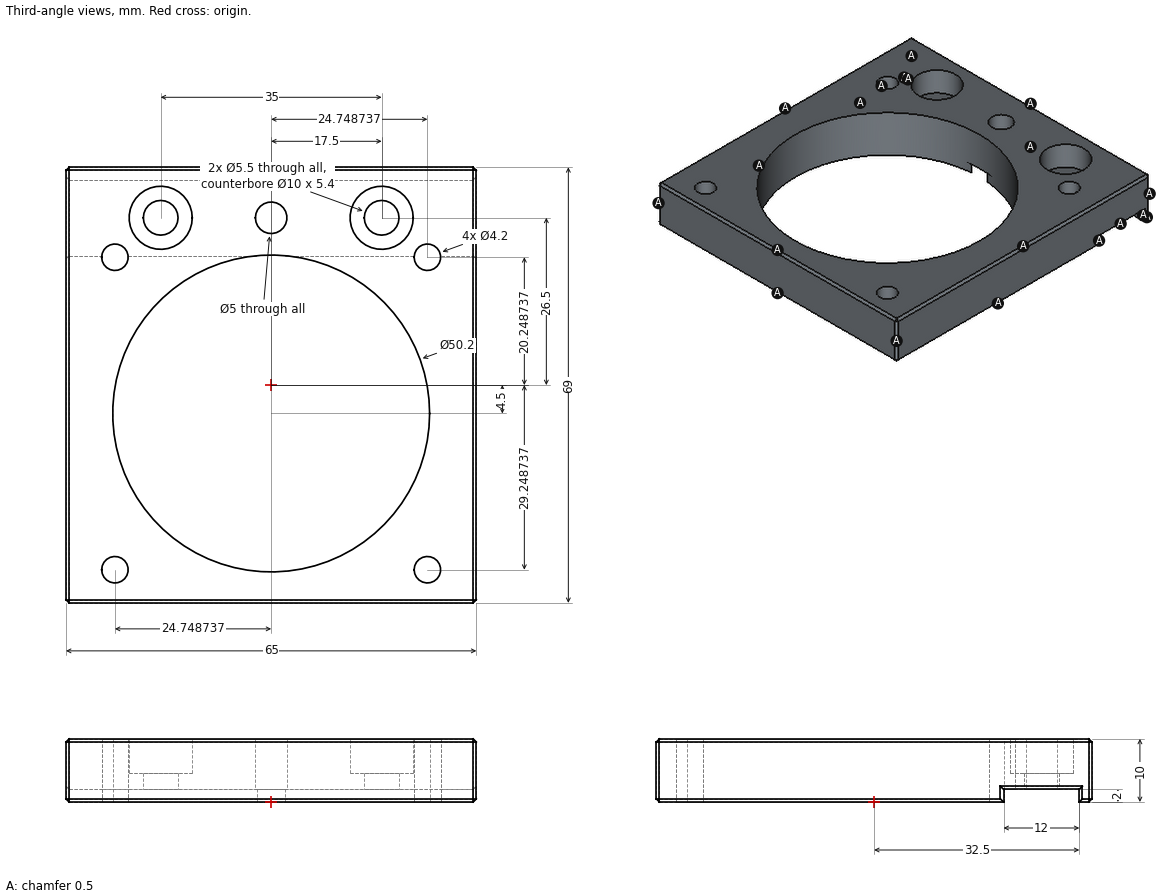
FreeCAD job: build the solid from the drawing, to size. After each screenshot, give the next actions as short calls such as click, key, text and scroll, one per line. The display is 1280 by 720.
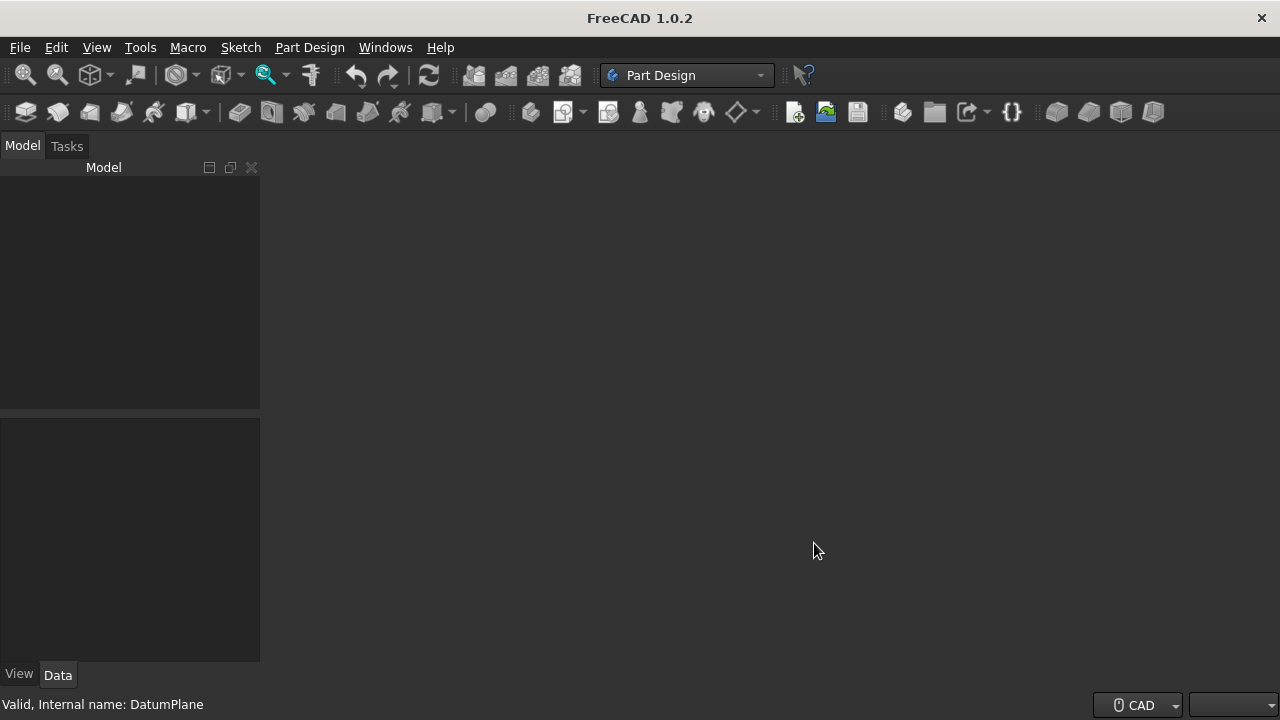
click(794, 112)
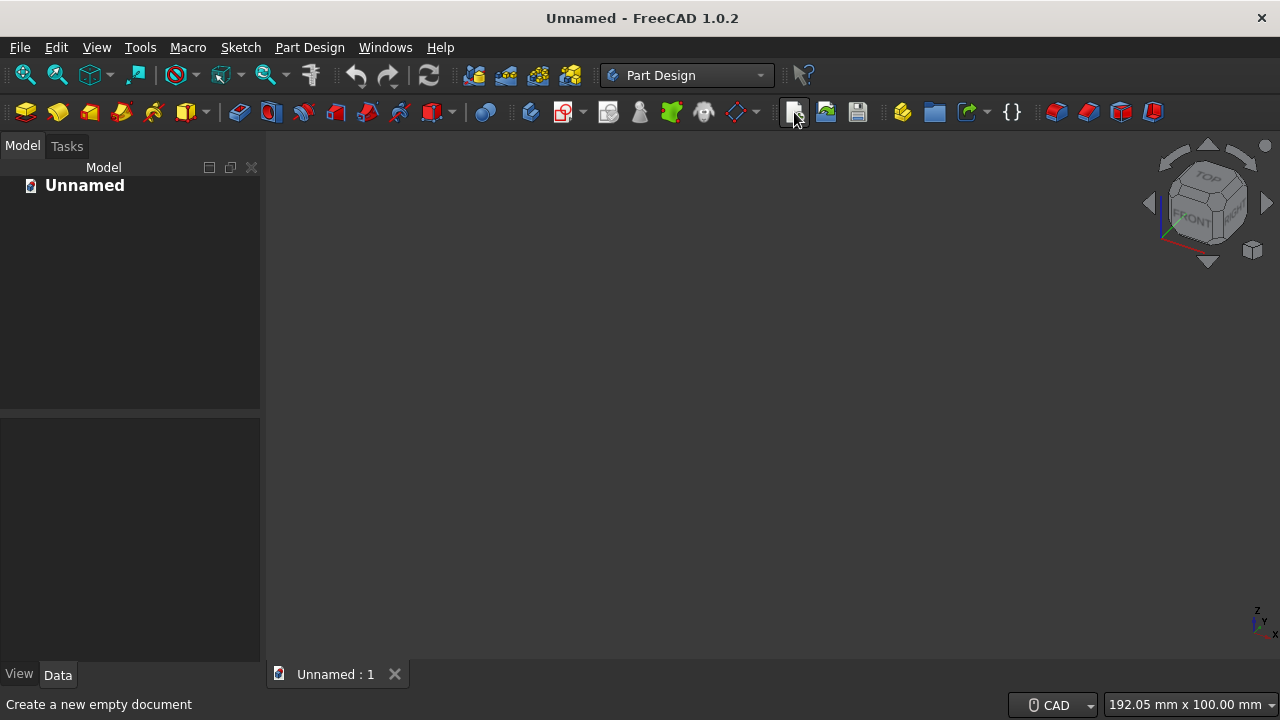
click(564, 112)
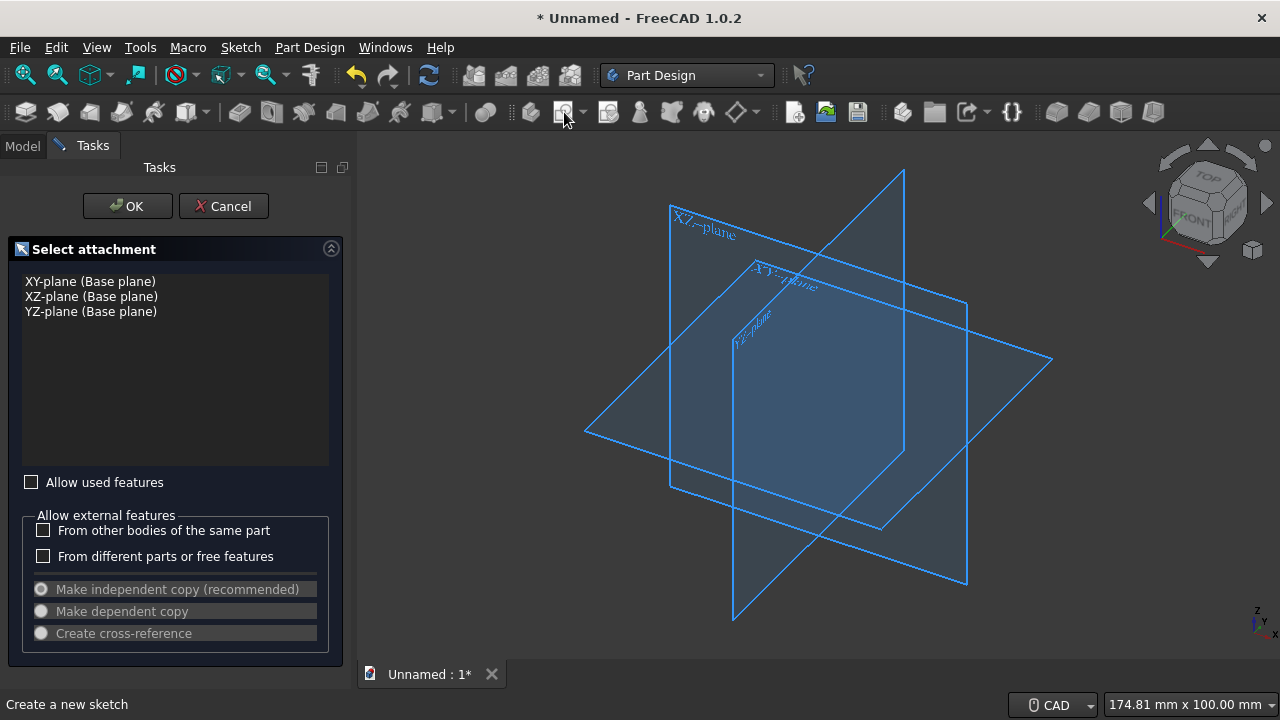
click(82, 282)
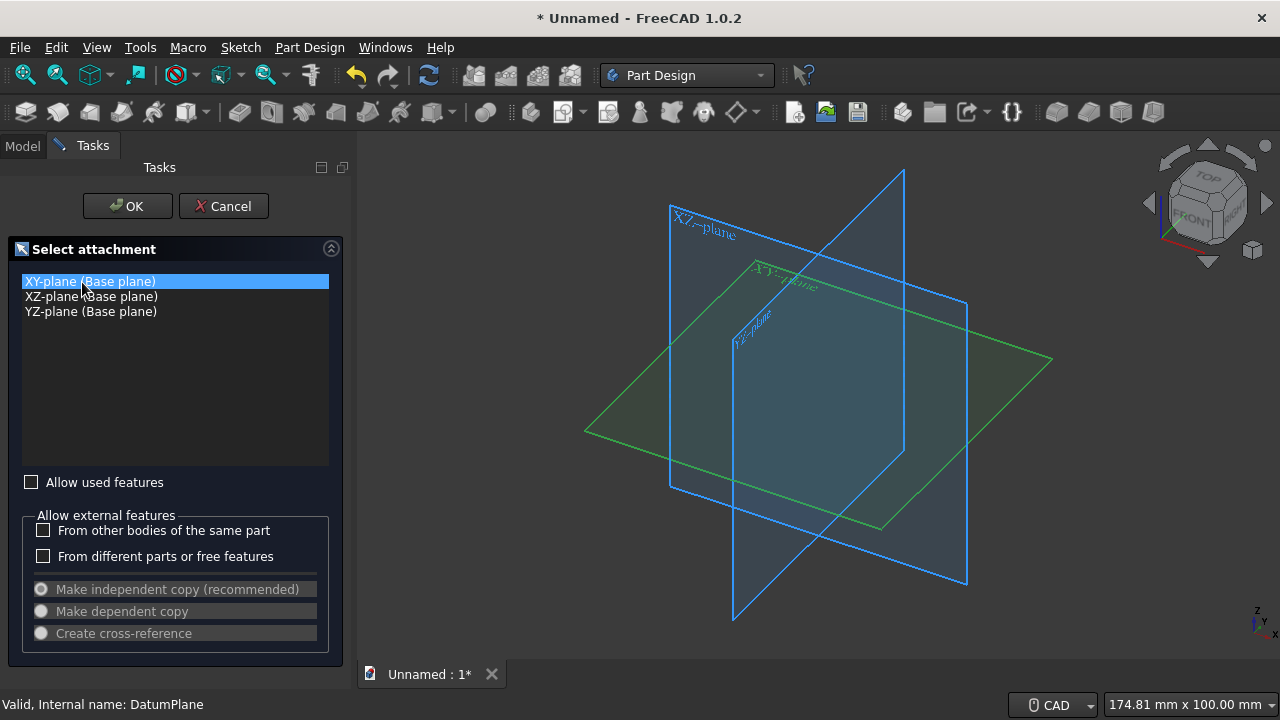
click(128, 206)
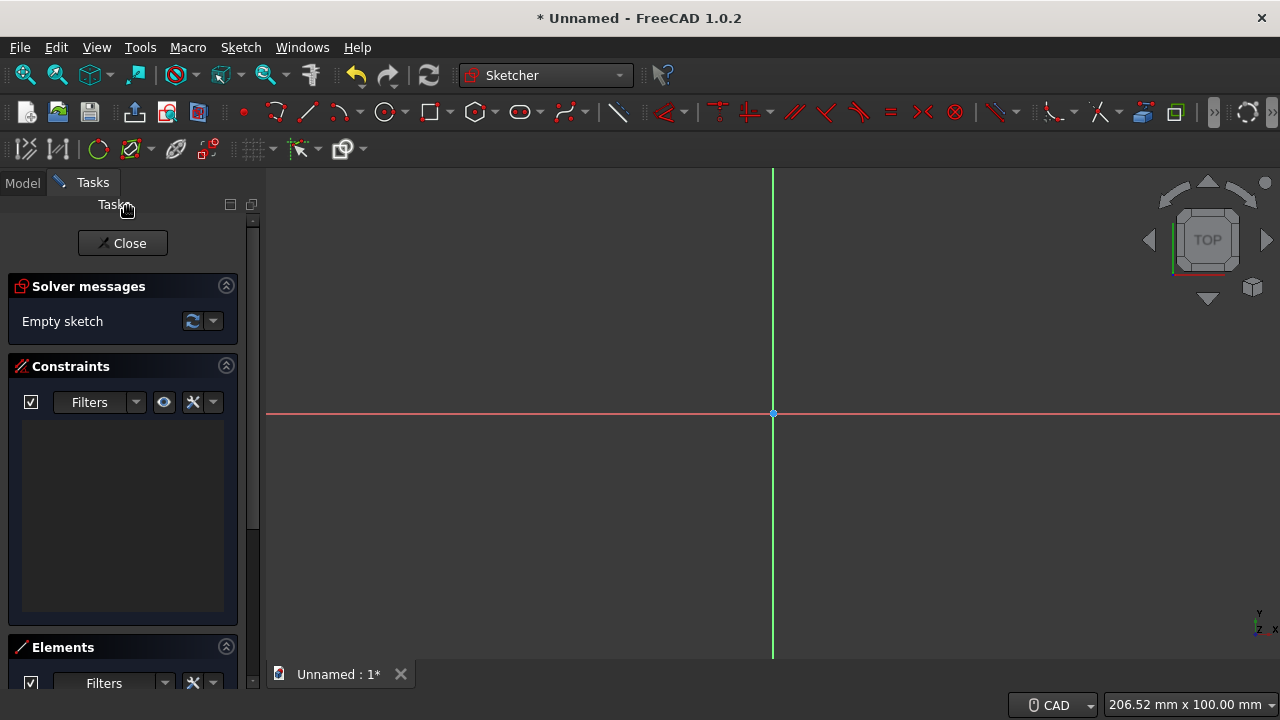
key(g)
key(v)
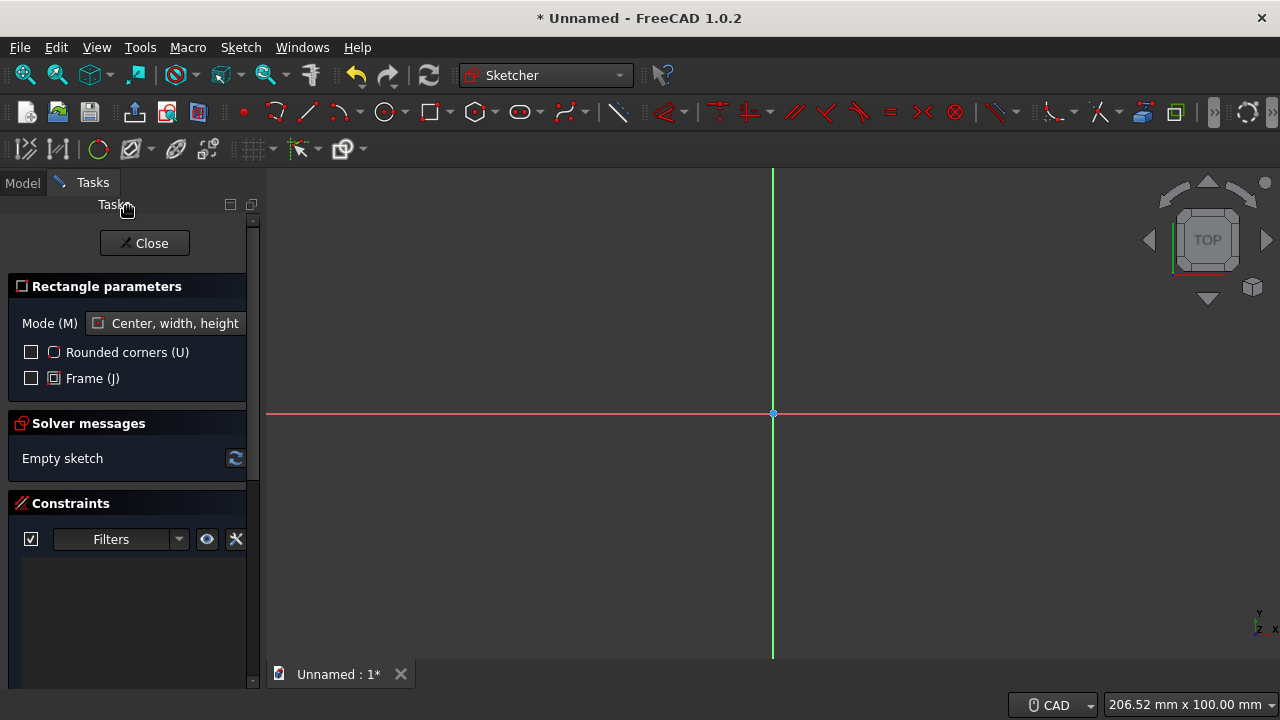
click(773, 414)
click(933, 244)
key(Escape)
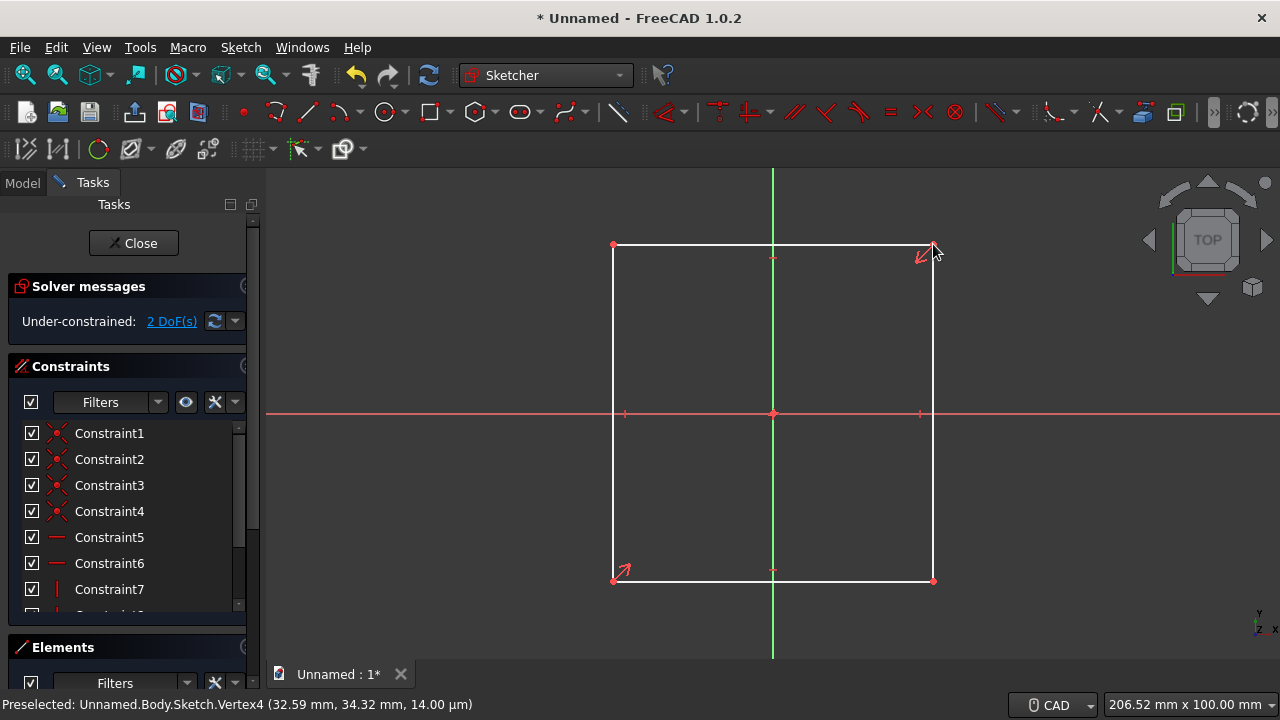
click(709, 582)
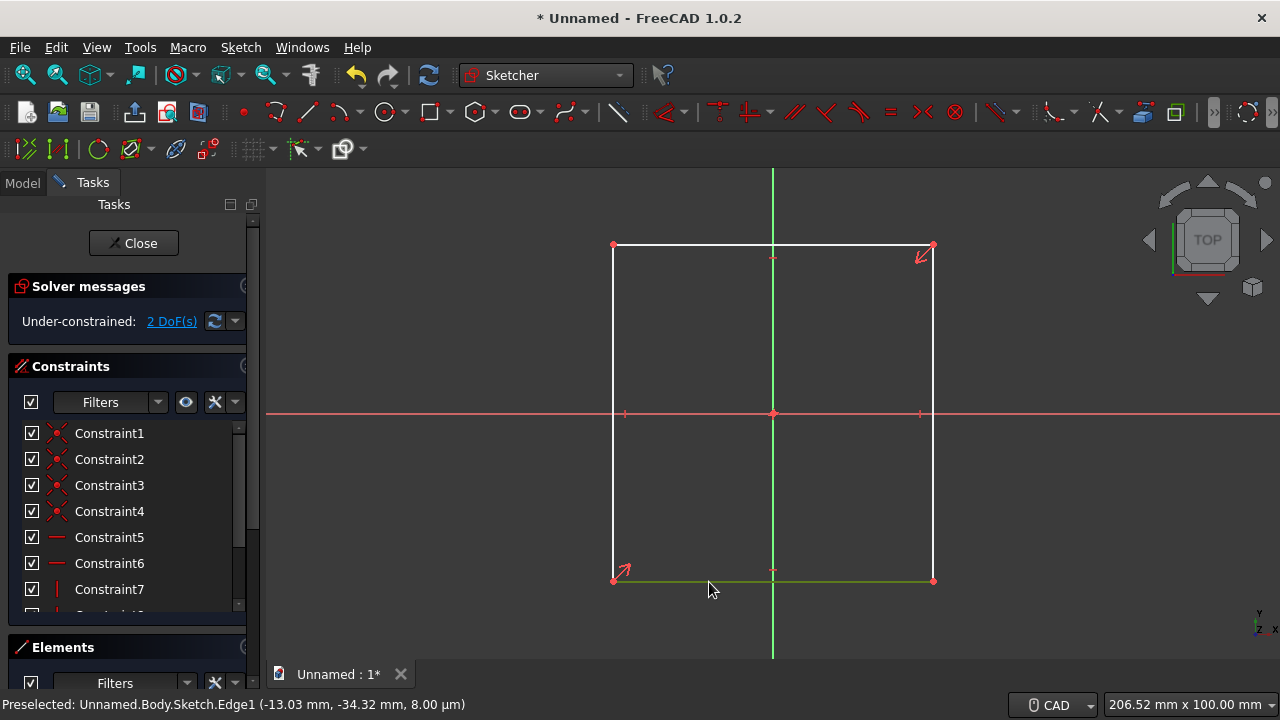
click(686, 112)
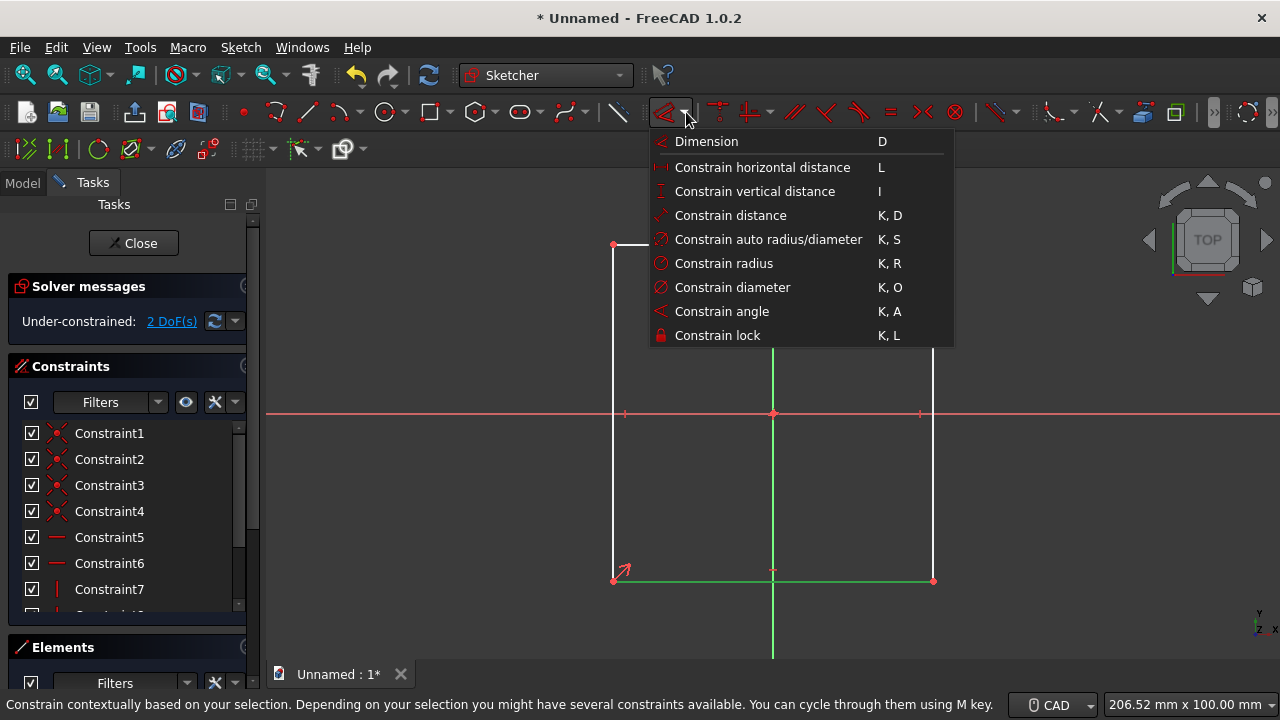
click(802, 167)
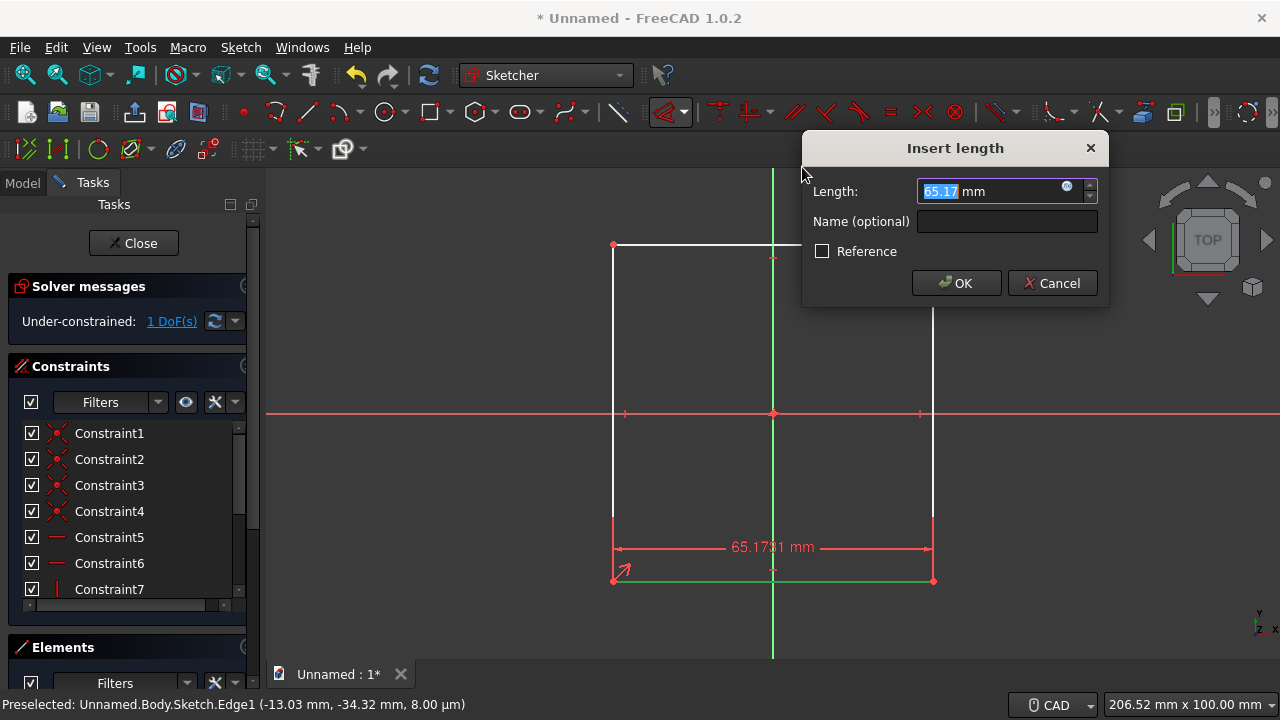
text(65)
key(Return)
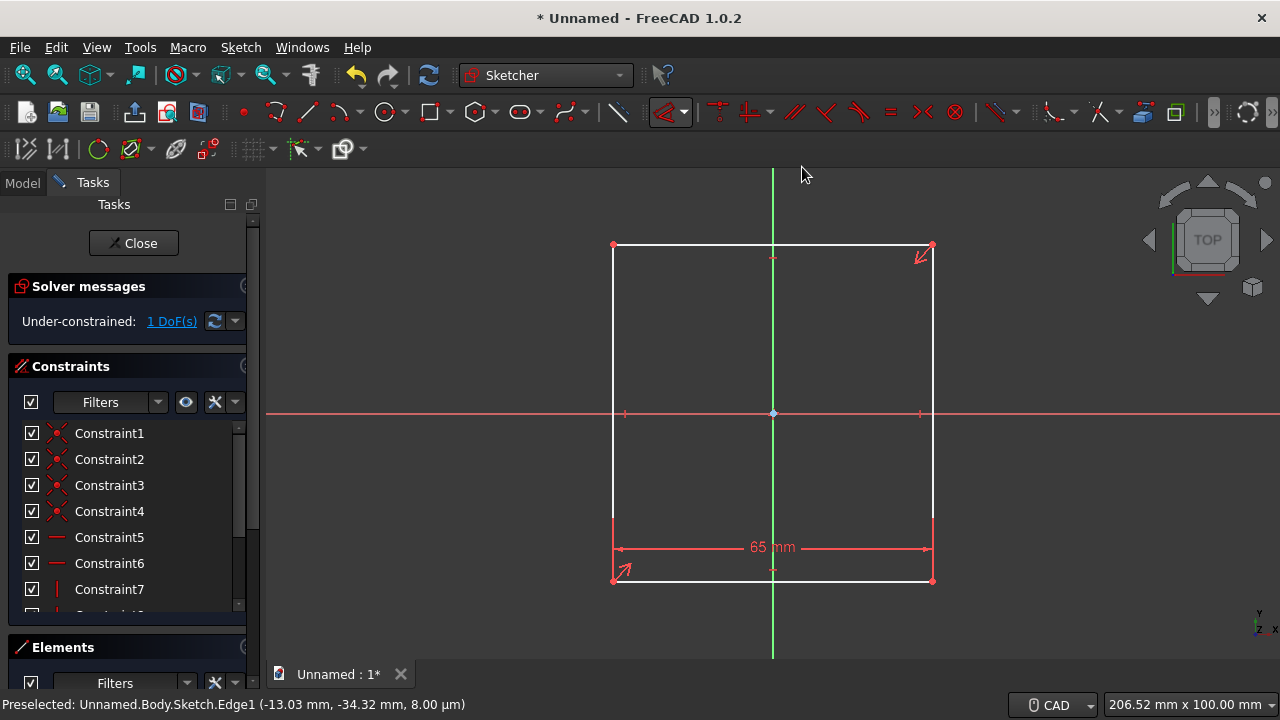
click(933, 481)